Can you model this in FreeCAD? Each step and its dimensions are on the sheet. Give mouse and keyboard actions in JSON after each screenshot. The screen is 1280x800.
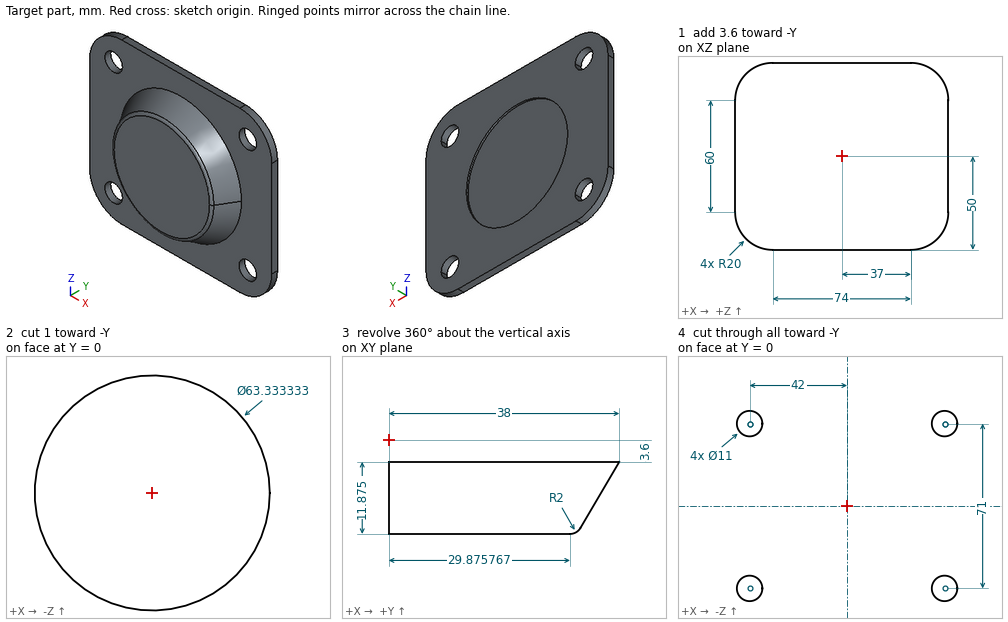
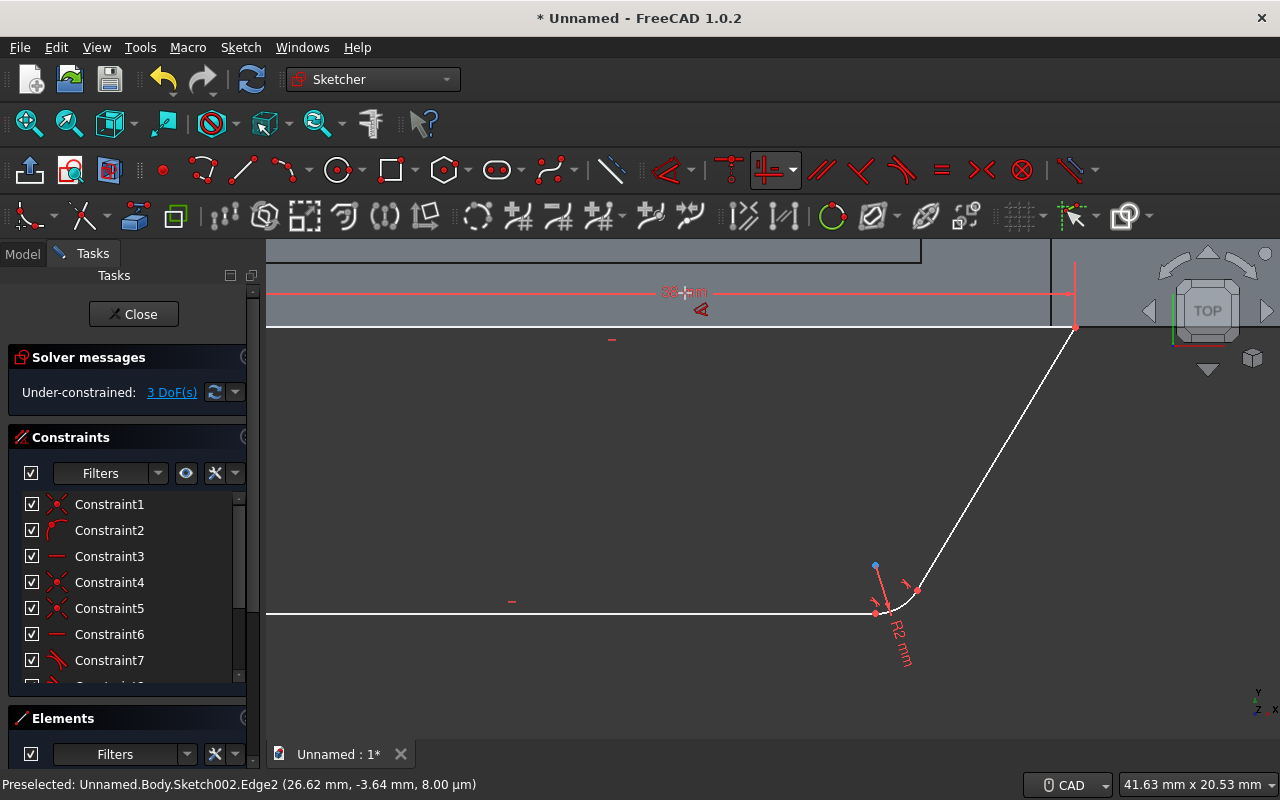
{"action": "left_click", "coordinate": [1075, 327]}
{"action": "left_click", "coordinate": [1109, 297]}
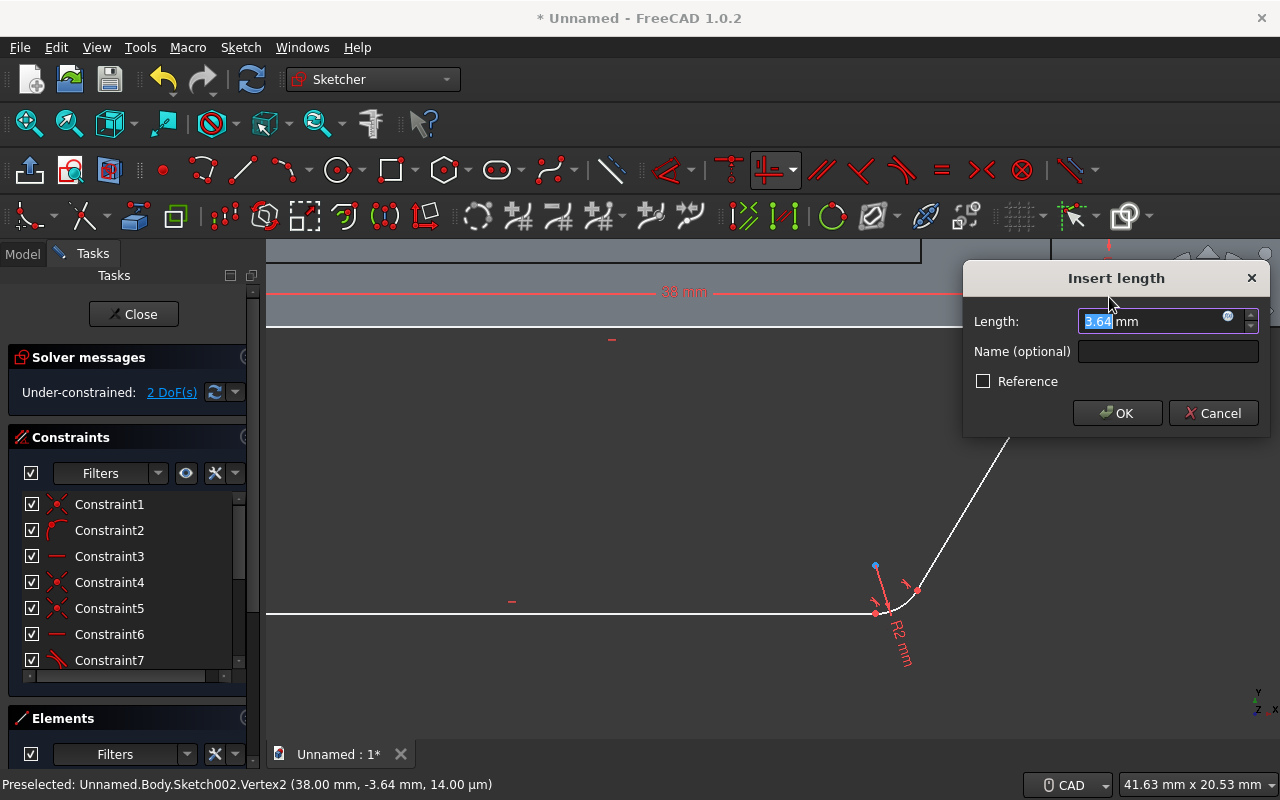
{"action": "type", "text": "3.6"}
{"action": "key", "text": "Return"}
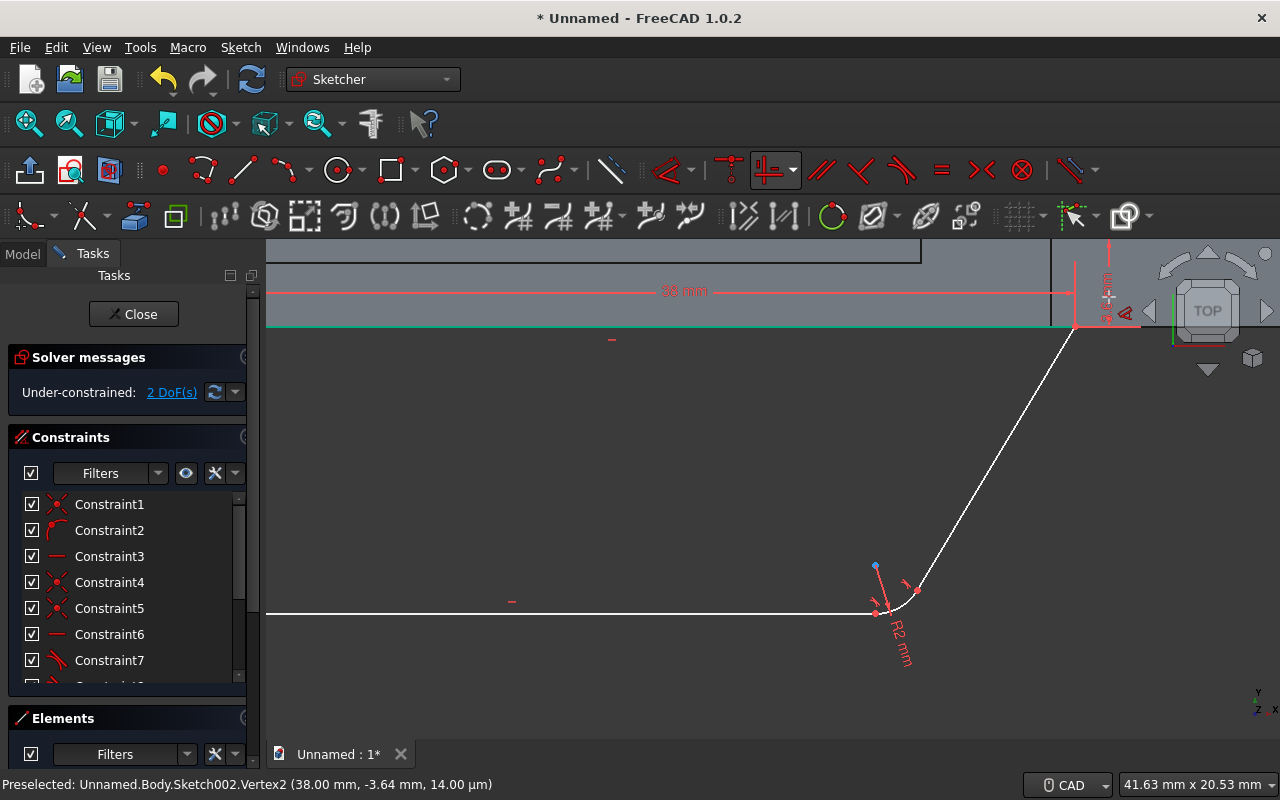
{"action": "scroll", "coordinate": [892, 614], "scroll_direction": "down", "scroll_amount": 2}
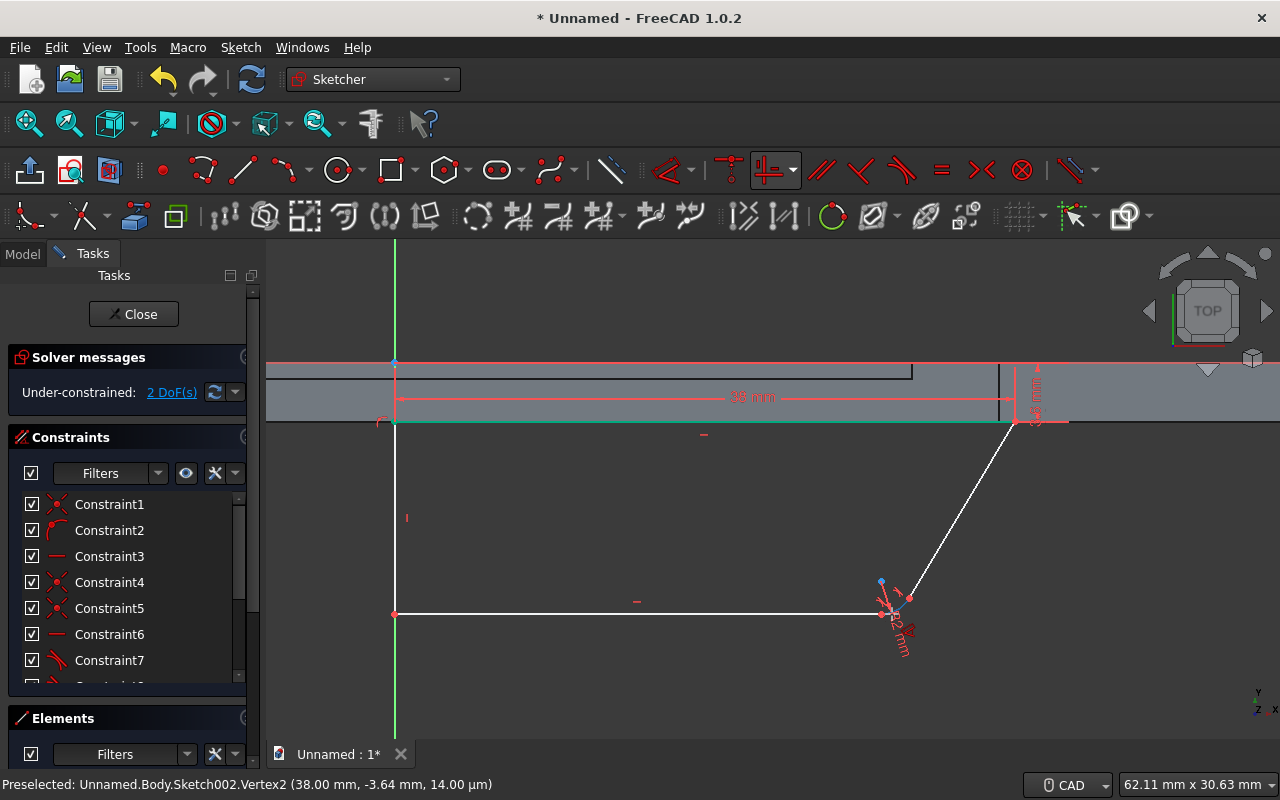
{"action": "left_click", "coordinate": [395, 479]}
{"action": "left_click", "coordinate": [361, 518]}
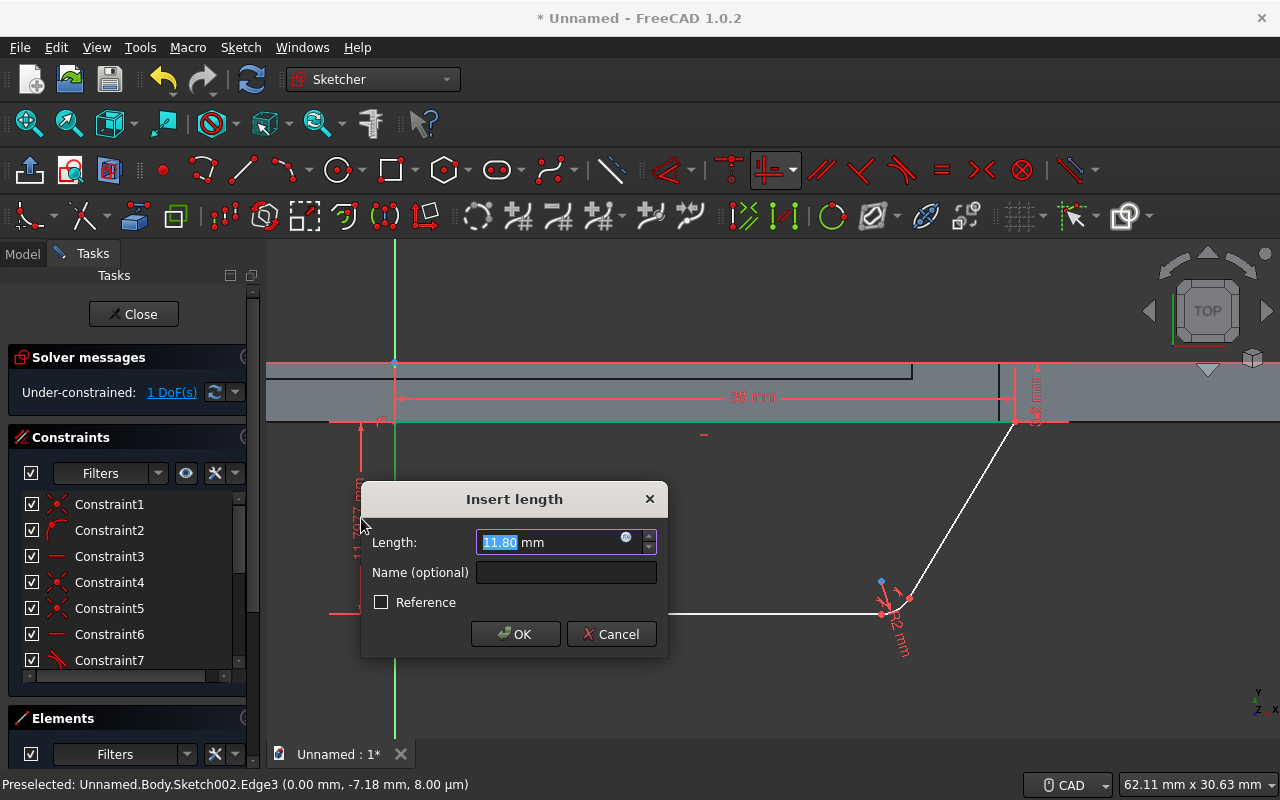
{"action": "type", "text": "11.875"}
{"action": "key", "text": "Return"}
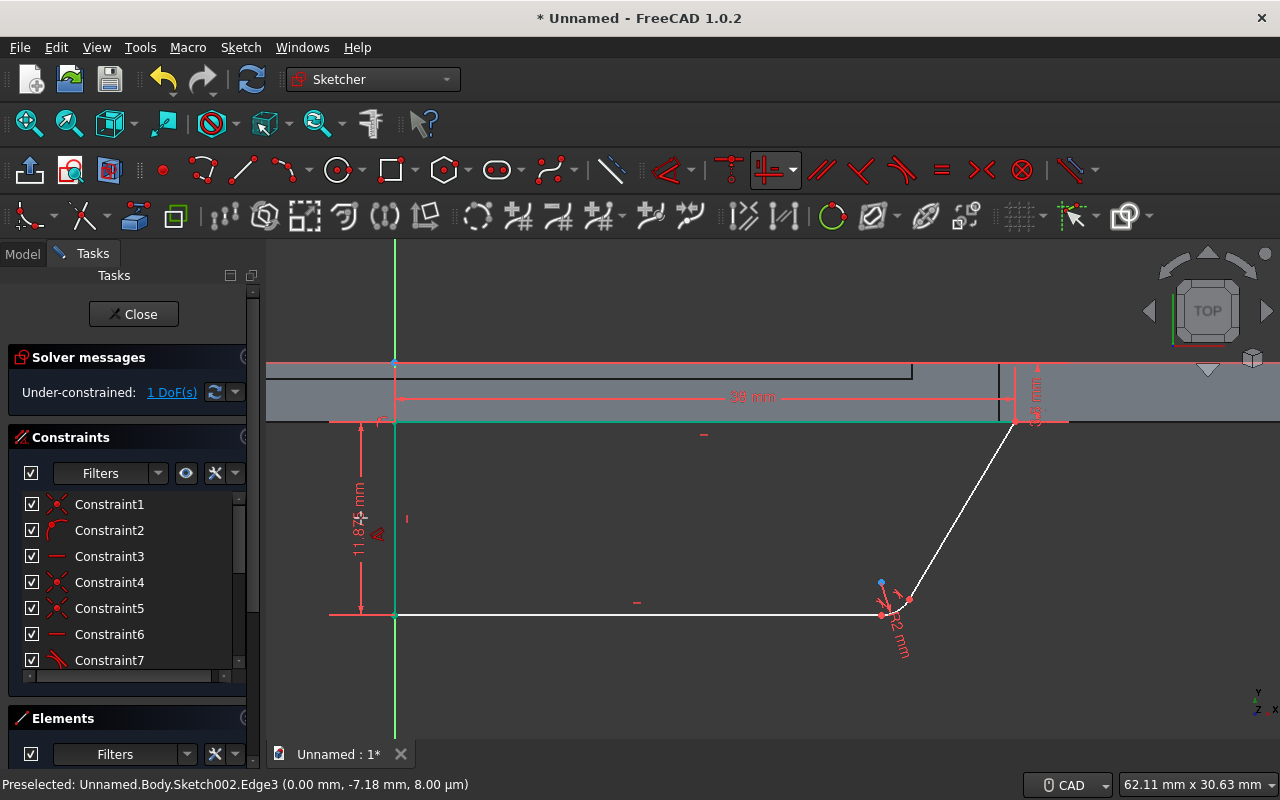
{"action": "left_click", "coordinate": [541, 615]}
{"action": "left_click", "coordinate": [638, 649]}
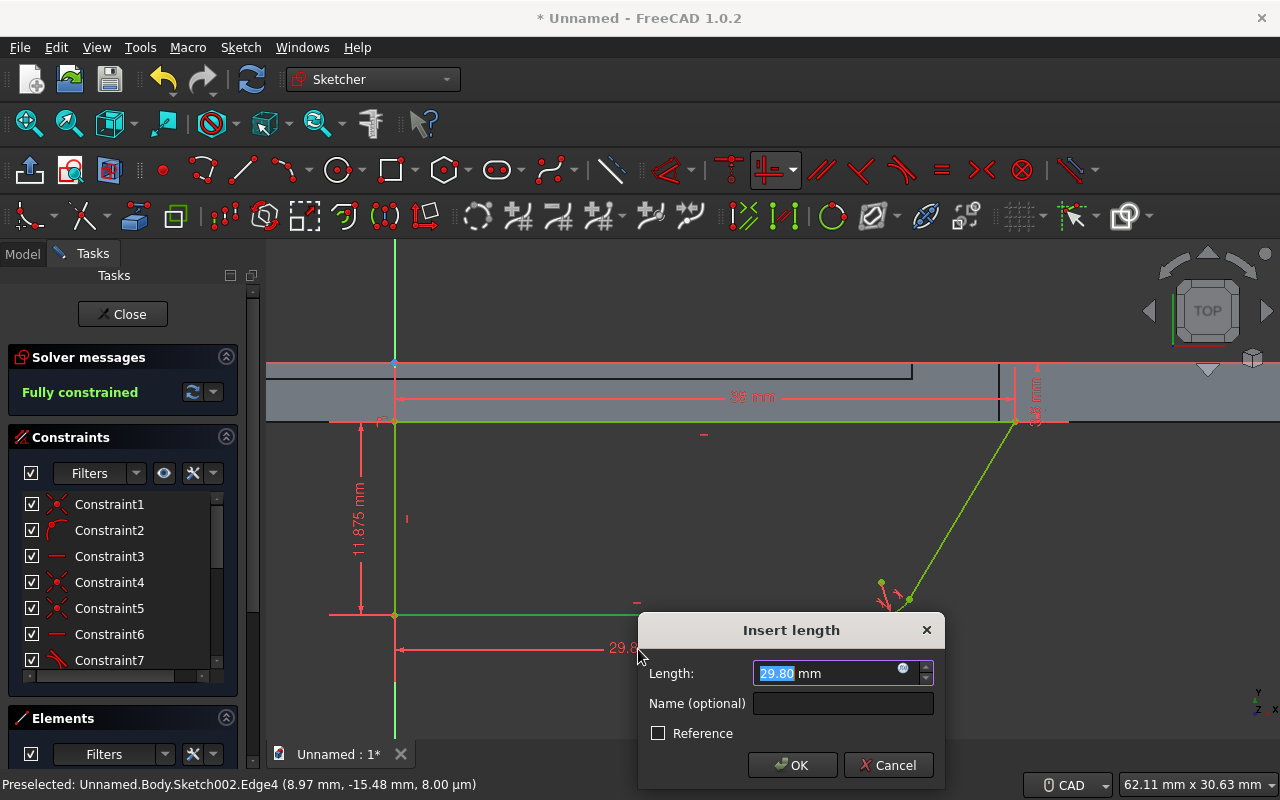
{"action": "type", "text": "29.875767"}
{"action": "key", "text": "Return"}
{"action": "key", "text": "Escape"}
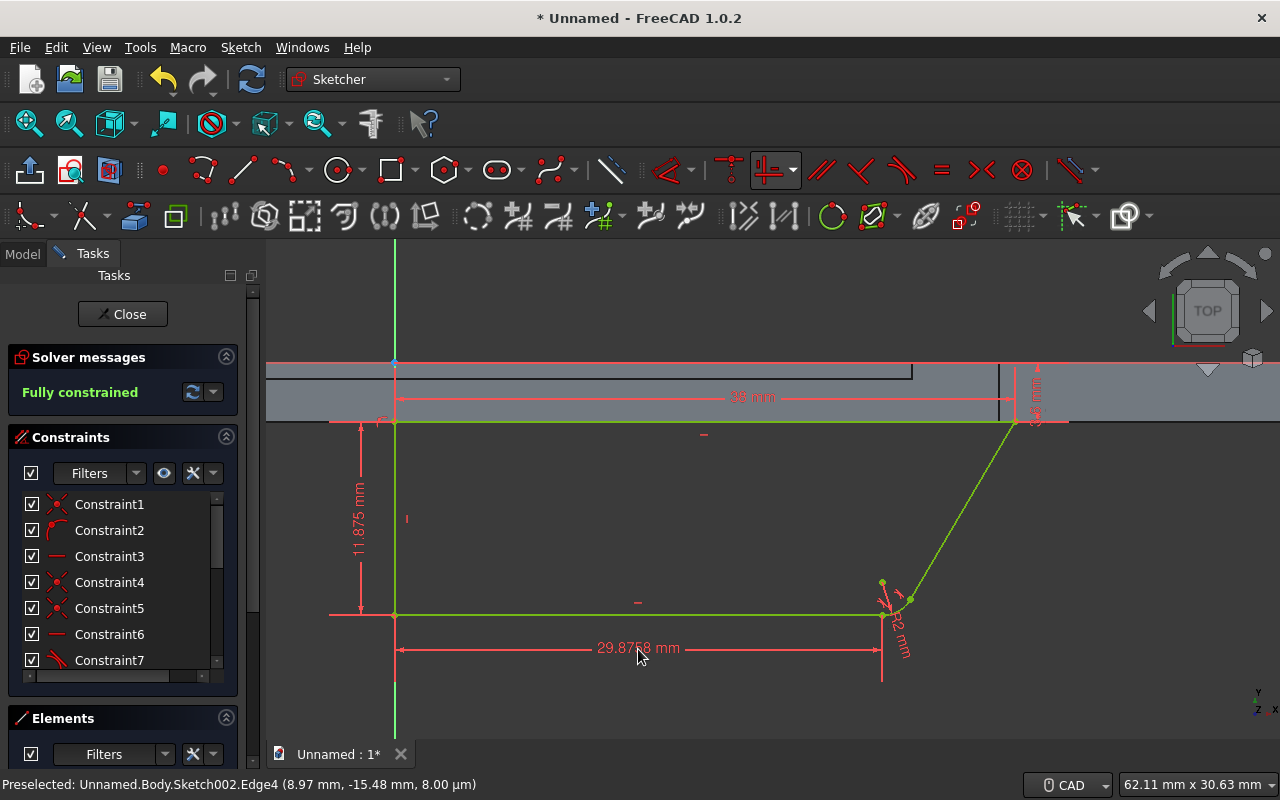
{"action": "left_click", "coordinate": [123, 314]}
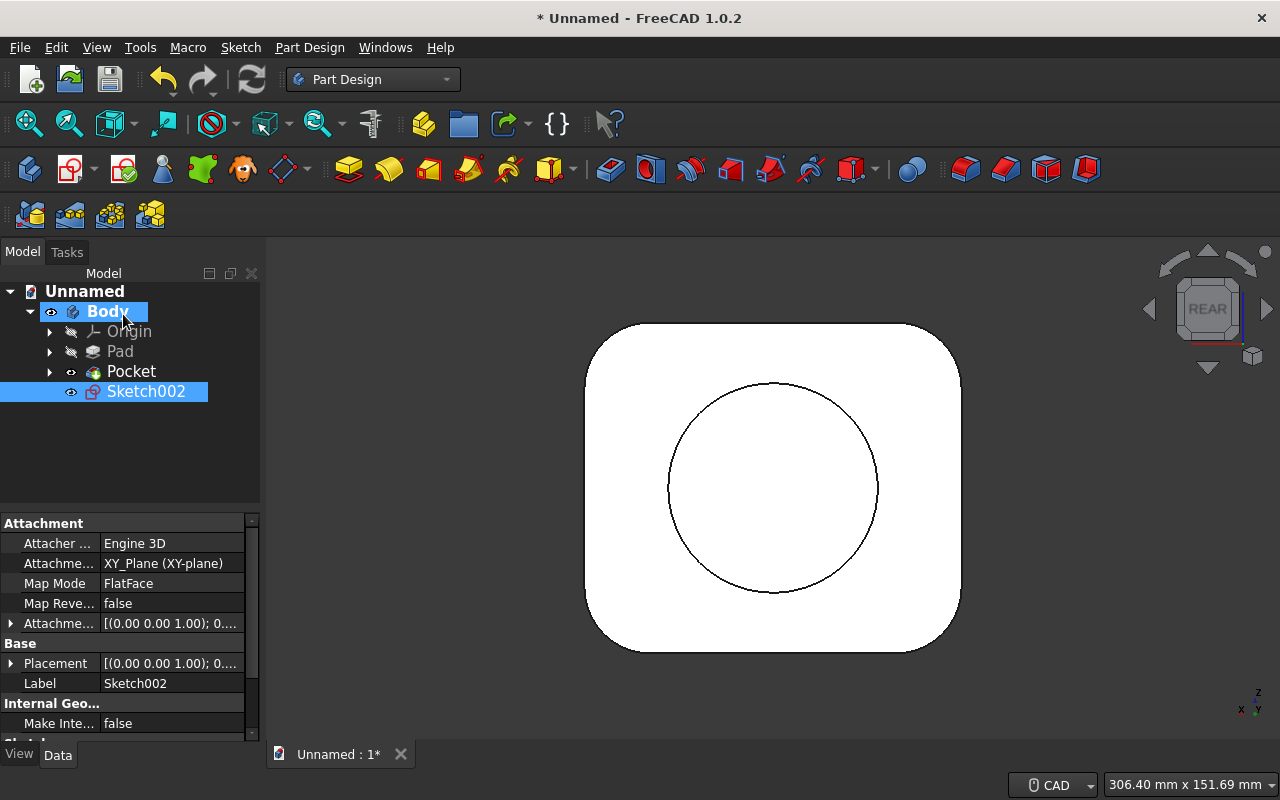
{"action": "left_click", "coordinate": [390, 170]}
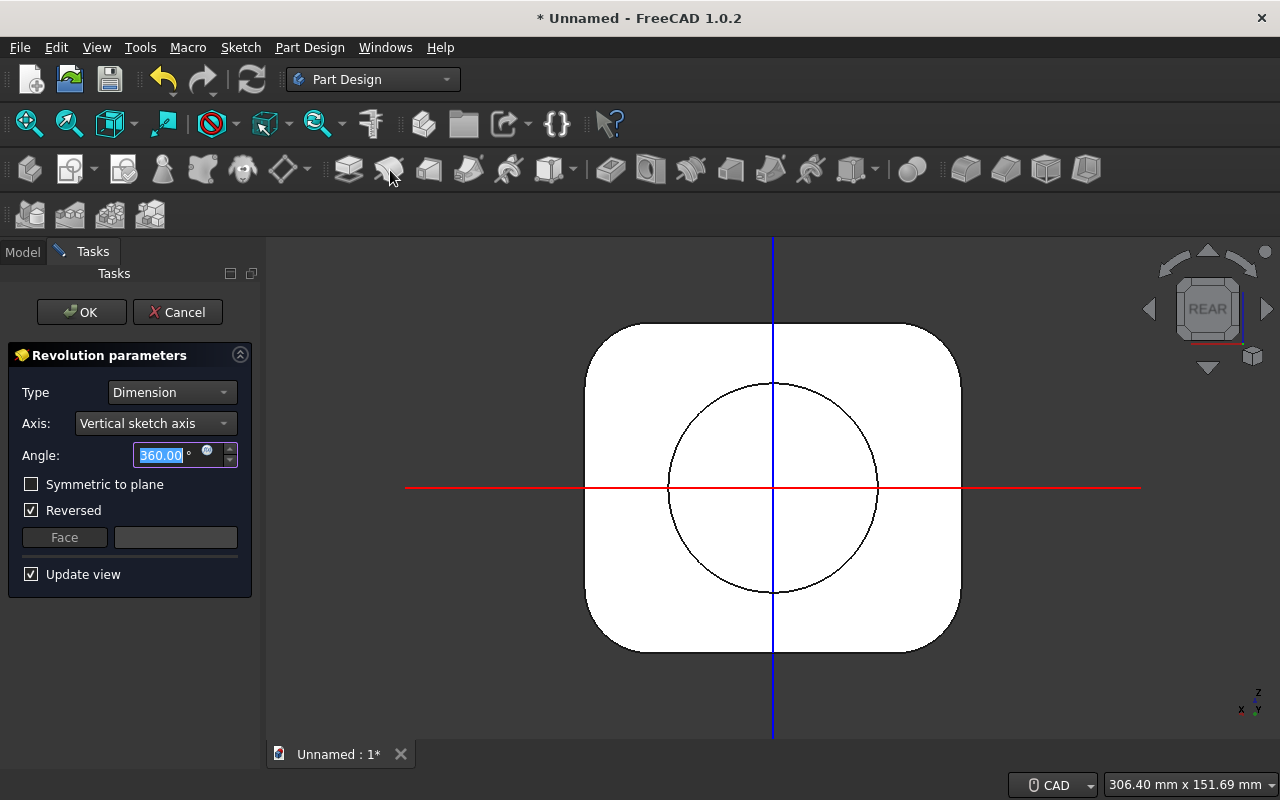
{"action": "left_click", "coordinate": [82, 312]}